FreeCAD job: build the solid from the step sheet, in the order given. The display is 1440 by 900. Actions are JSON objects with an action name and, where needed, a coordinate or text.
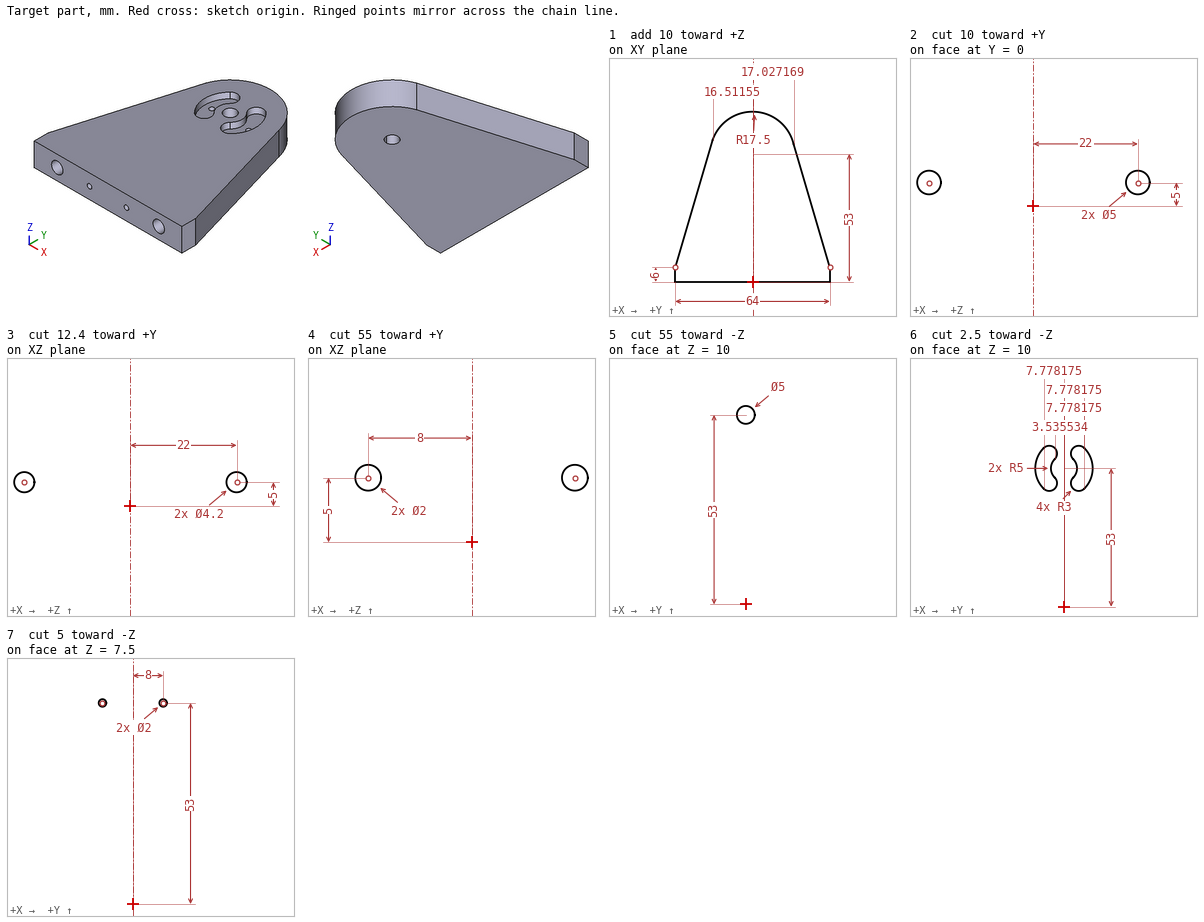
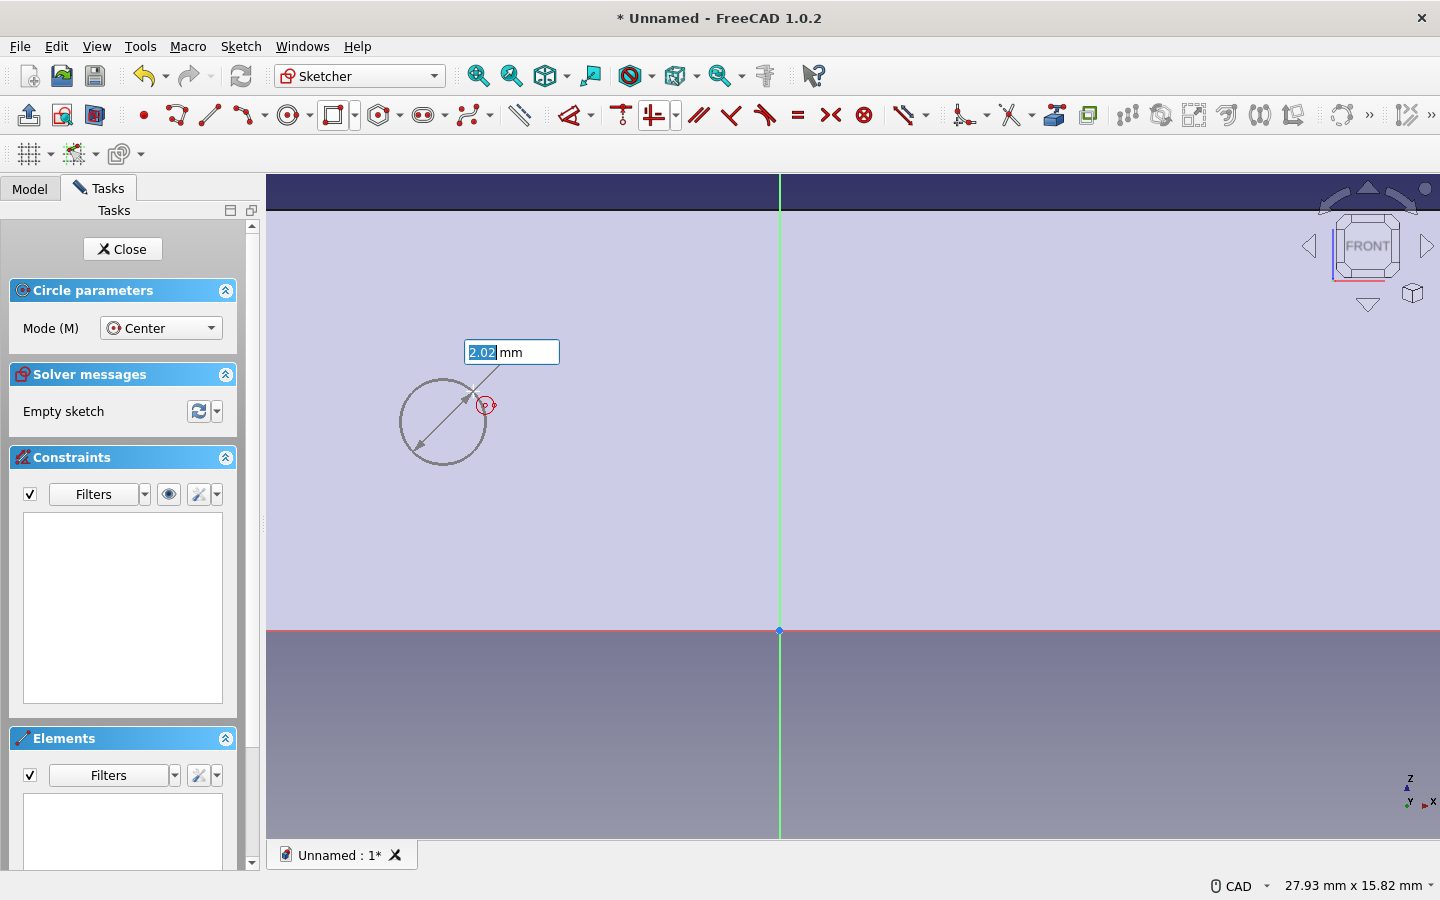
{"action": "type", "text": "2"}
{"action": "key", "text": "Return"}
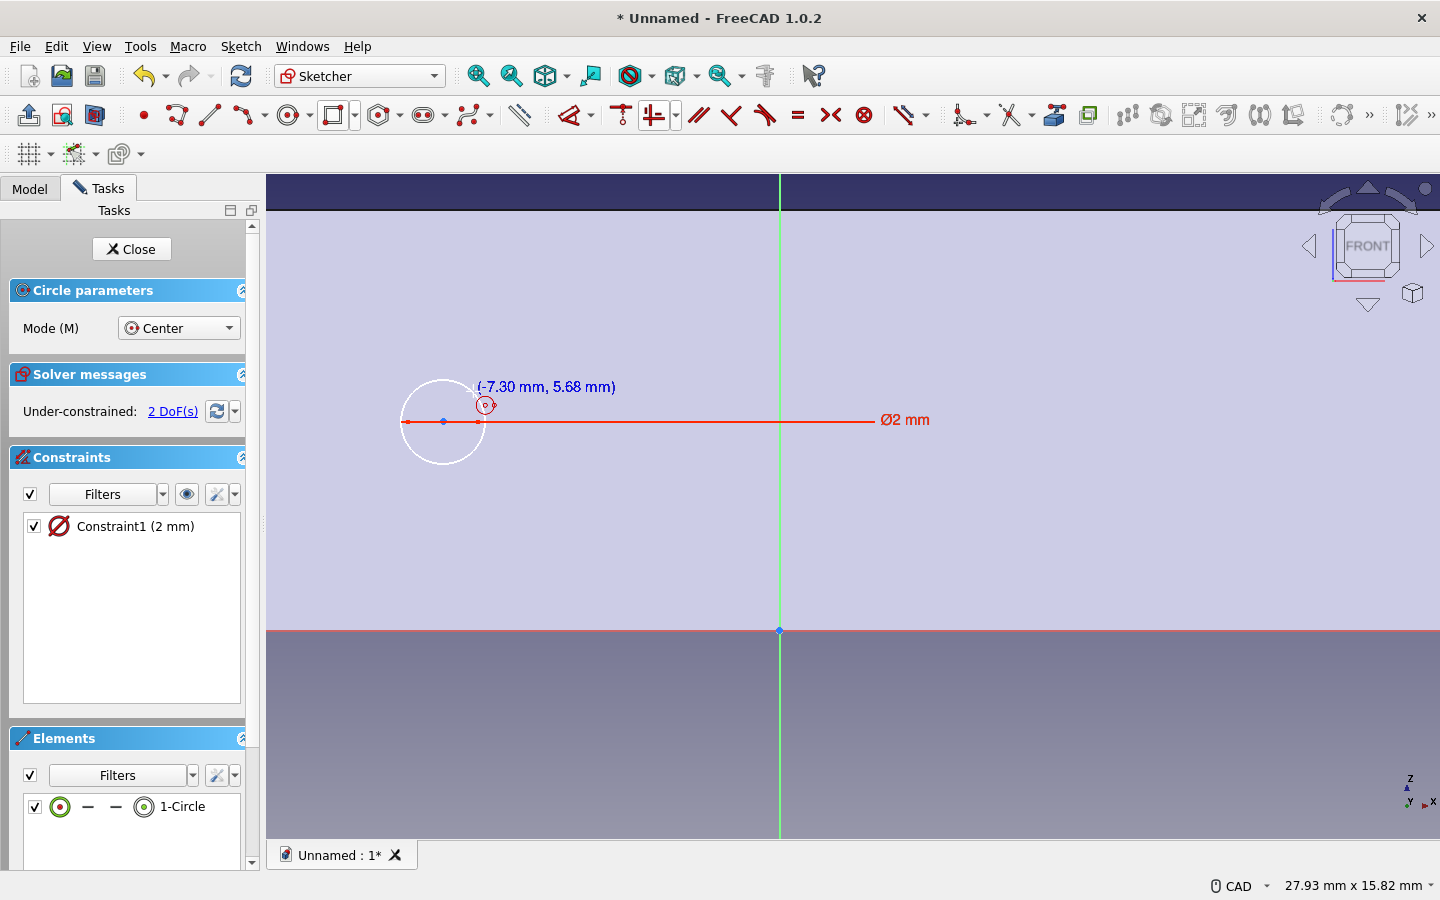
{"action": "left_click", "coordinate": [1116, 421]}
{"action": "mouse_move", "coordinate": [1146, 391]}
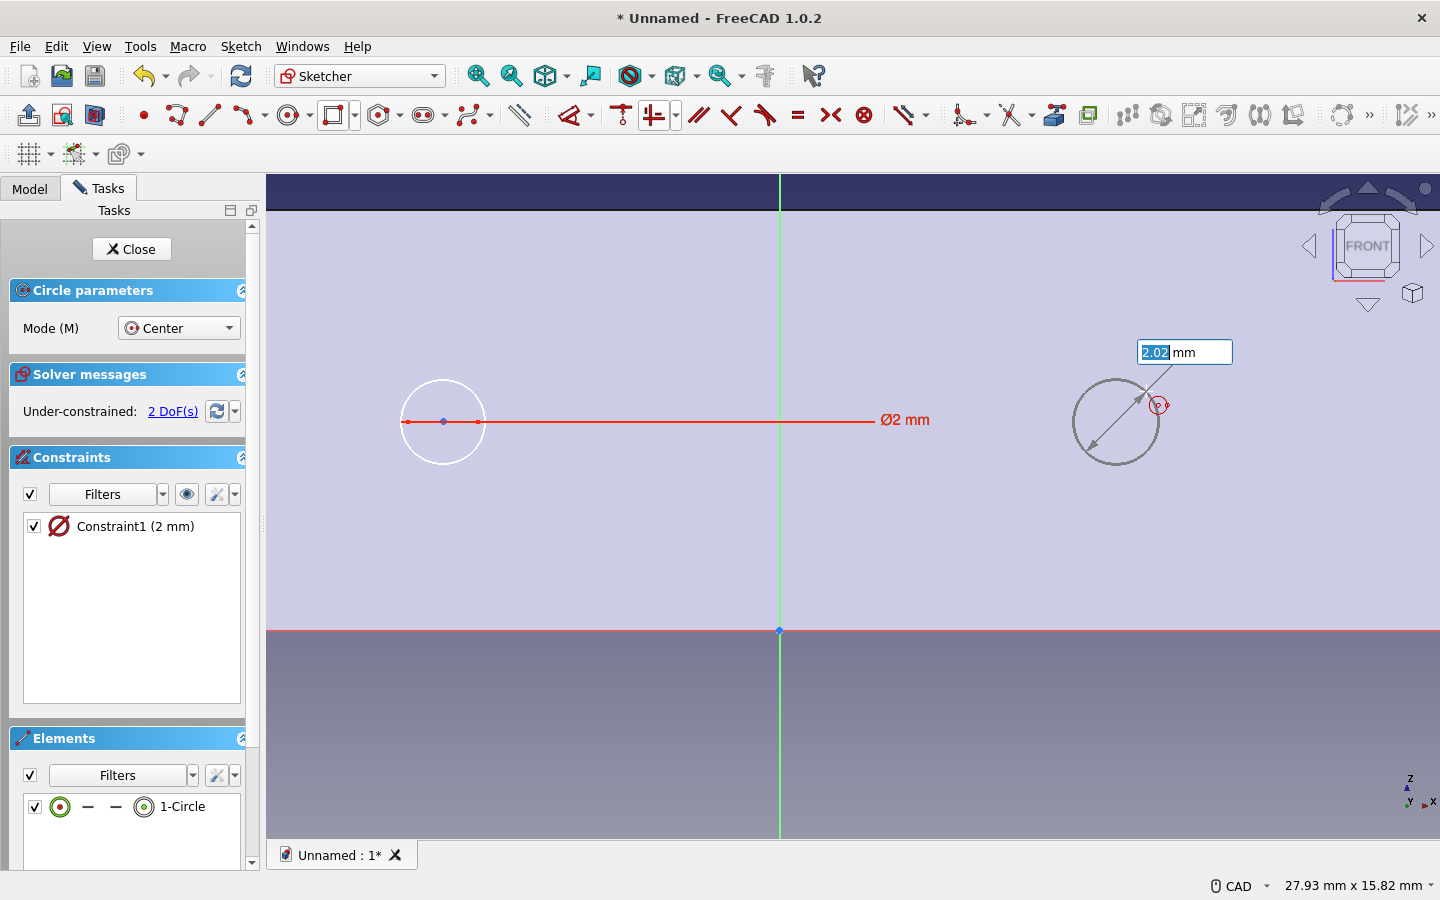
{"action": "type", "text": "2"}
{"action": "key", "text": "Return"}
{"action": "key", "text": "Escape"}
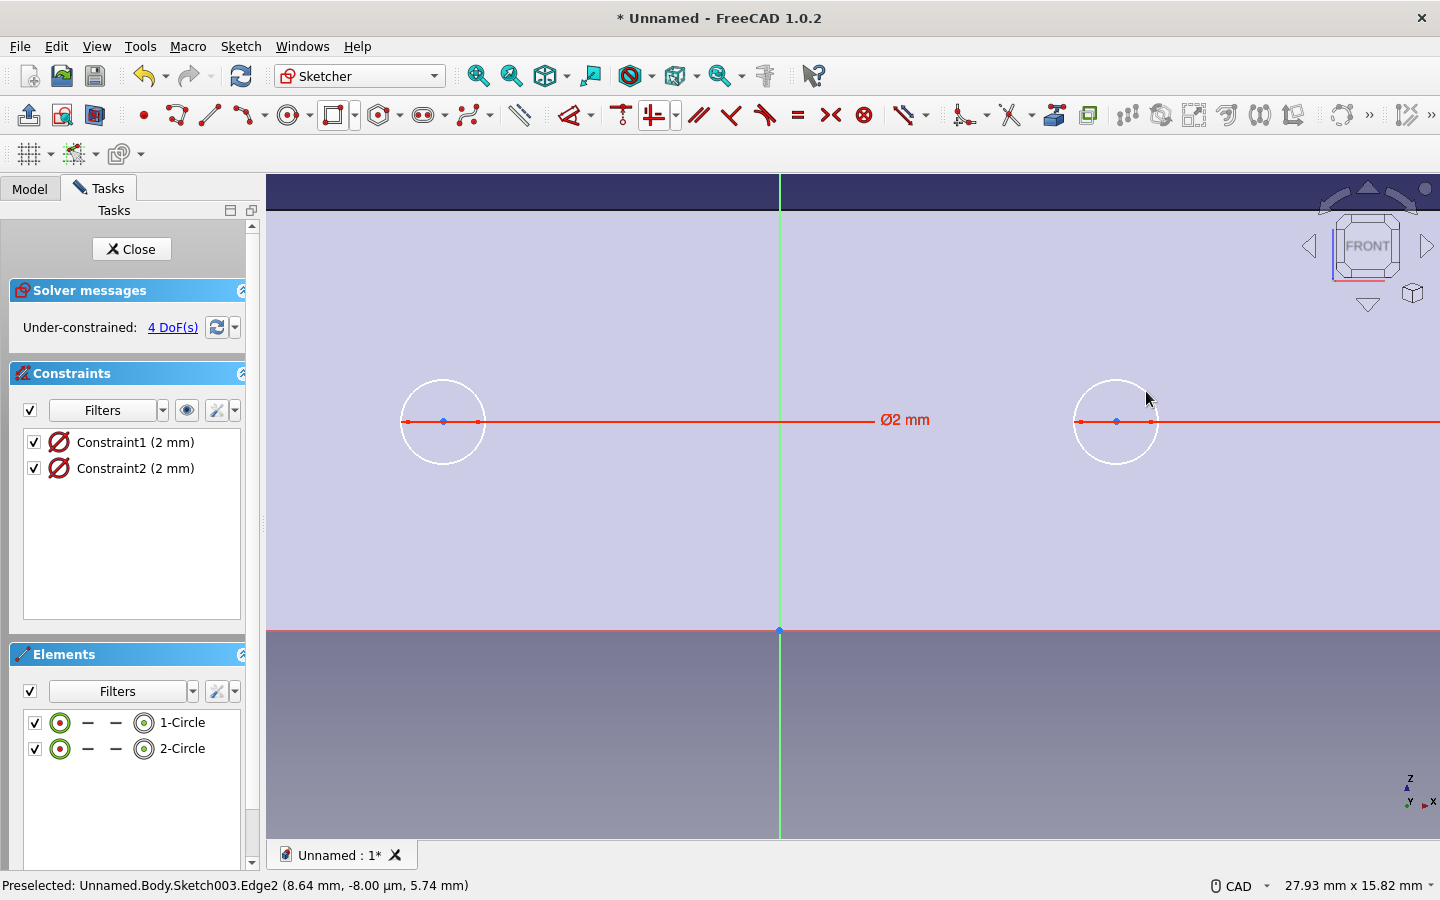
{"action": "left_click", "coordinate": [443, 422]}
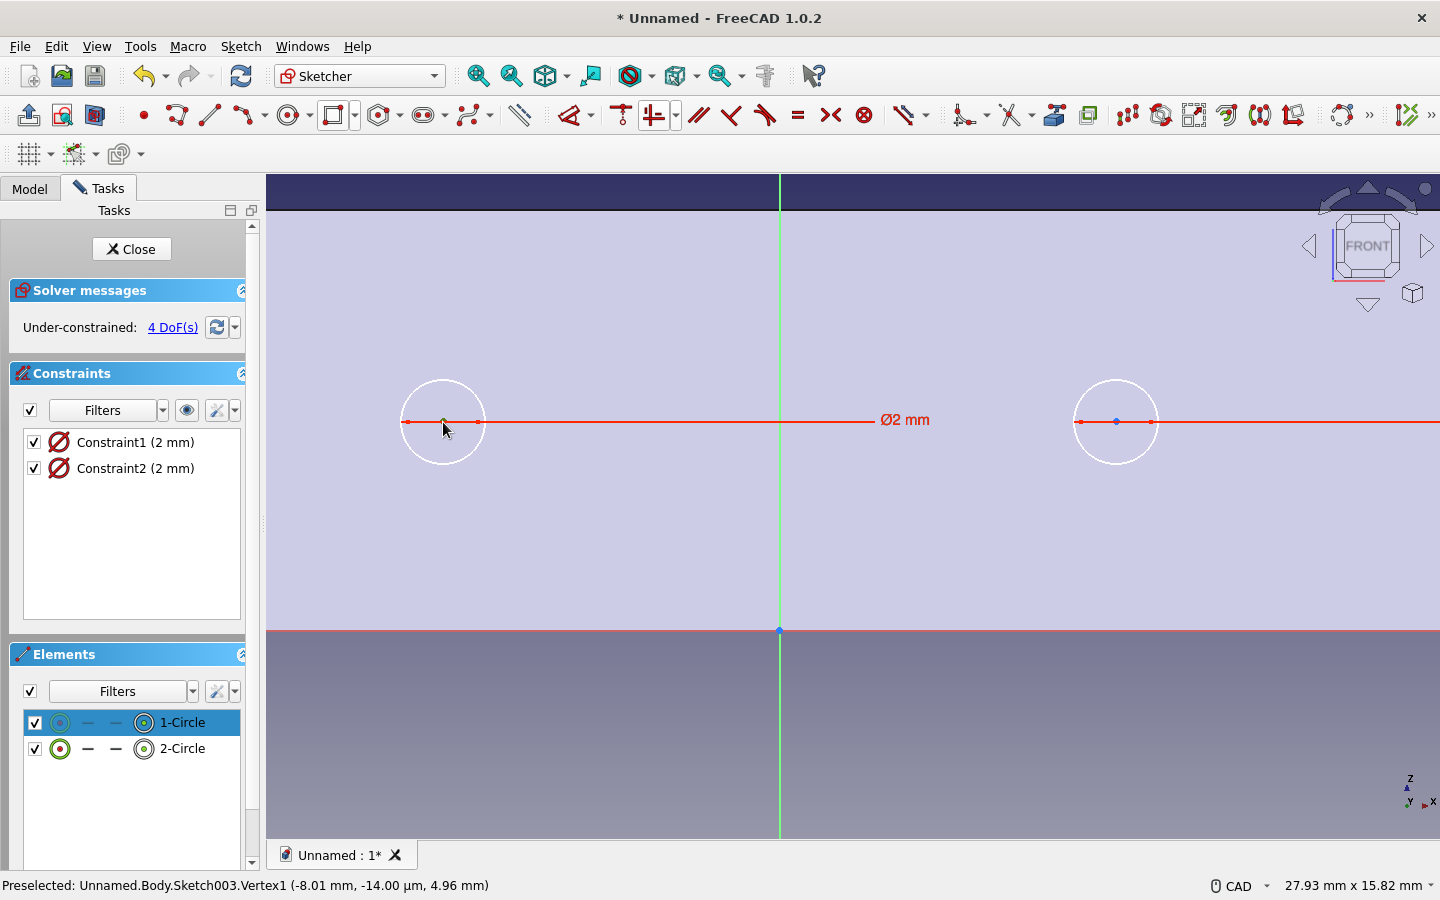
{"action": "left_click", "coordinate": [1116, 422]}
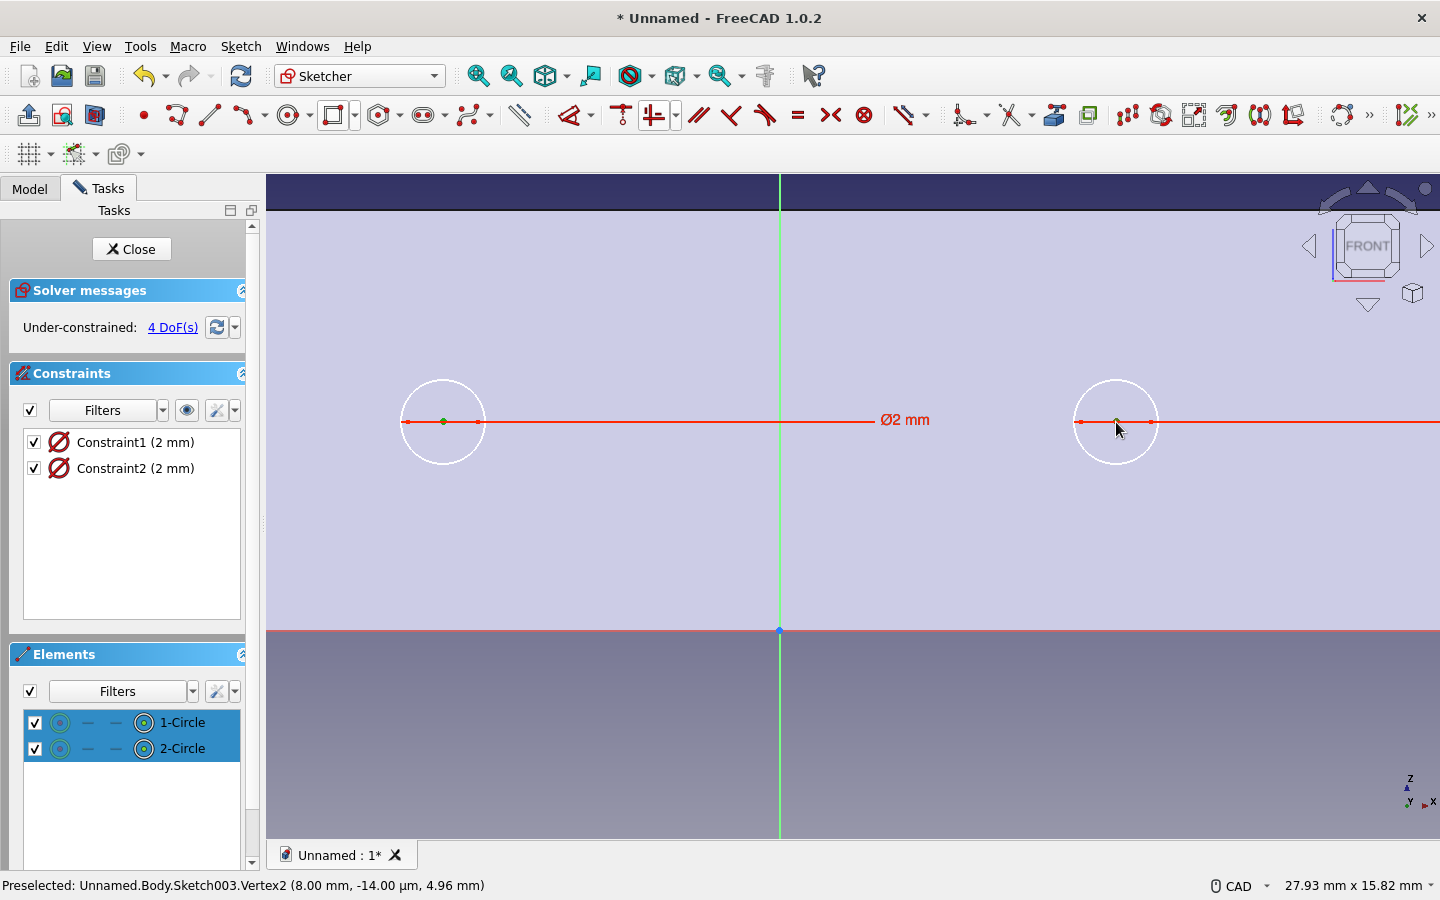
{"action": "left_click", "coordinate": [780, 768]}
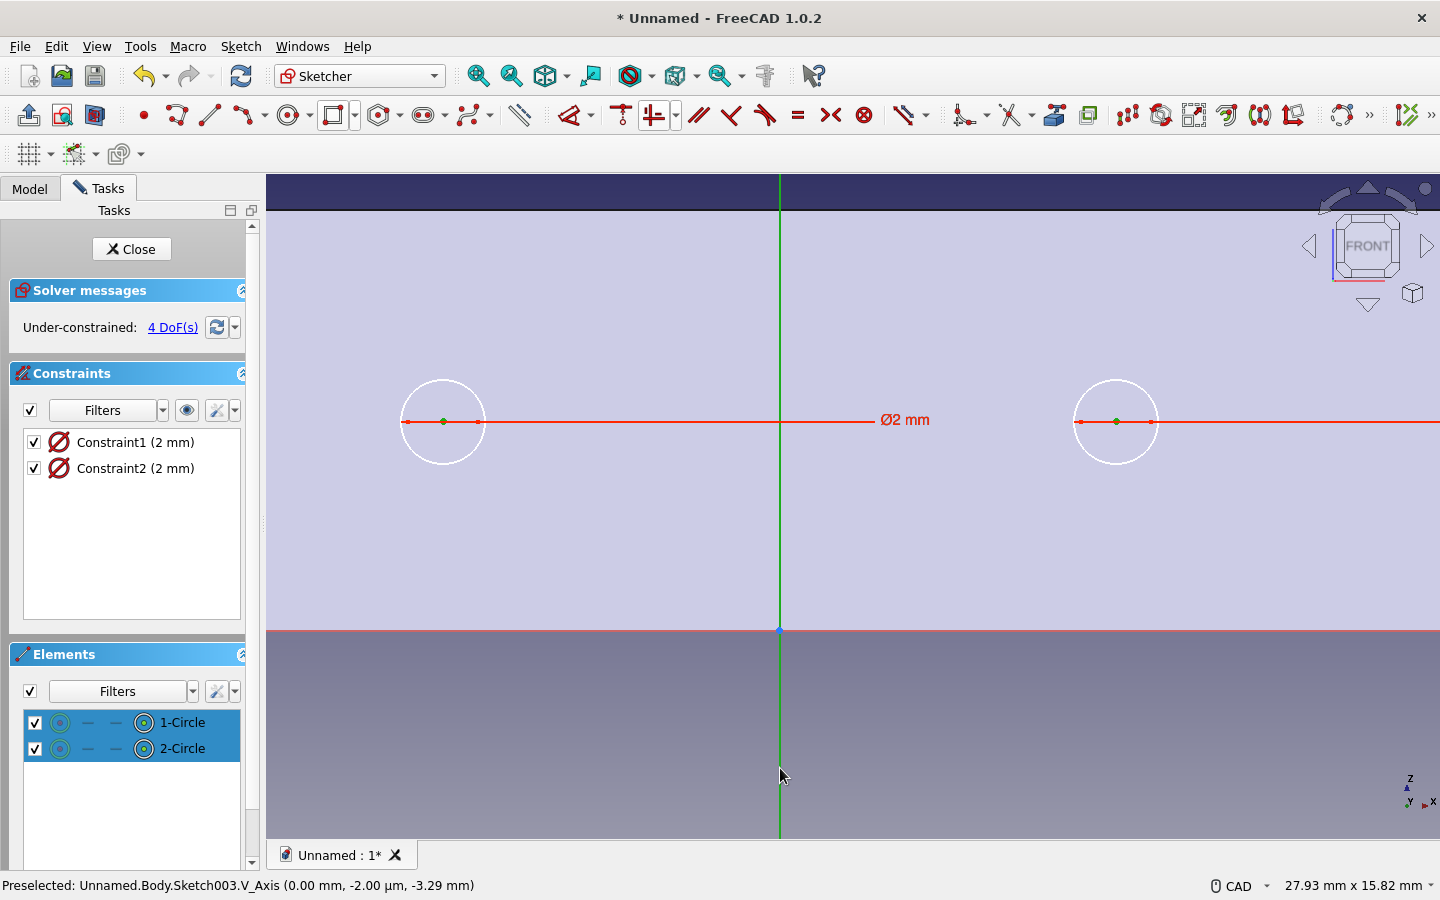
{"action": "left_click", "coordinate": [831, 116]}